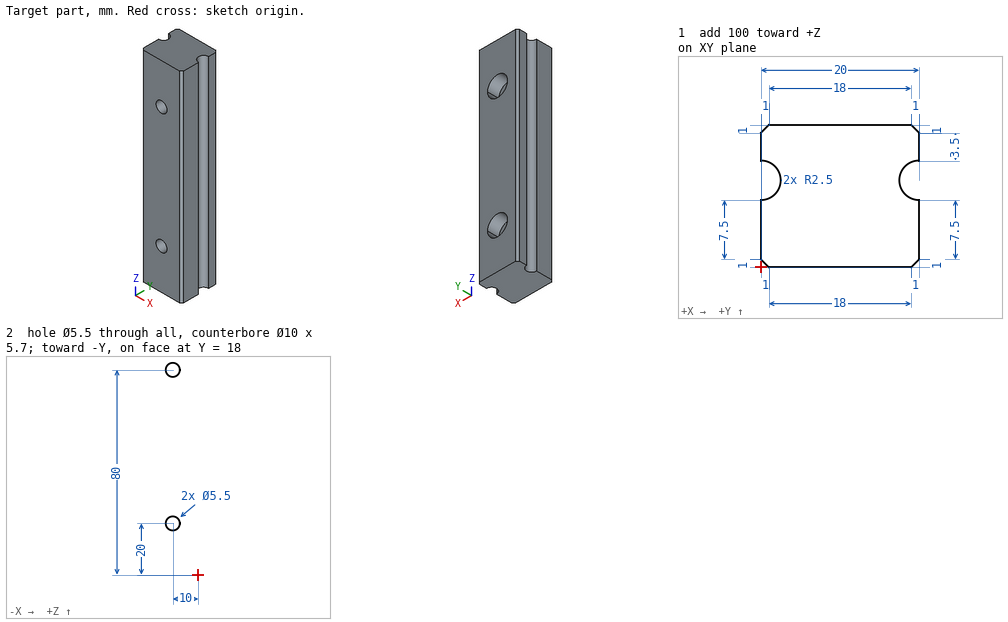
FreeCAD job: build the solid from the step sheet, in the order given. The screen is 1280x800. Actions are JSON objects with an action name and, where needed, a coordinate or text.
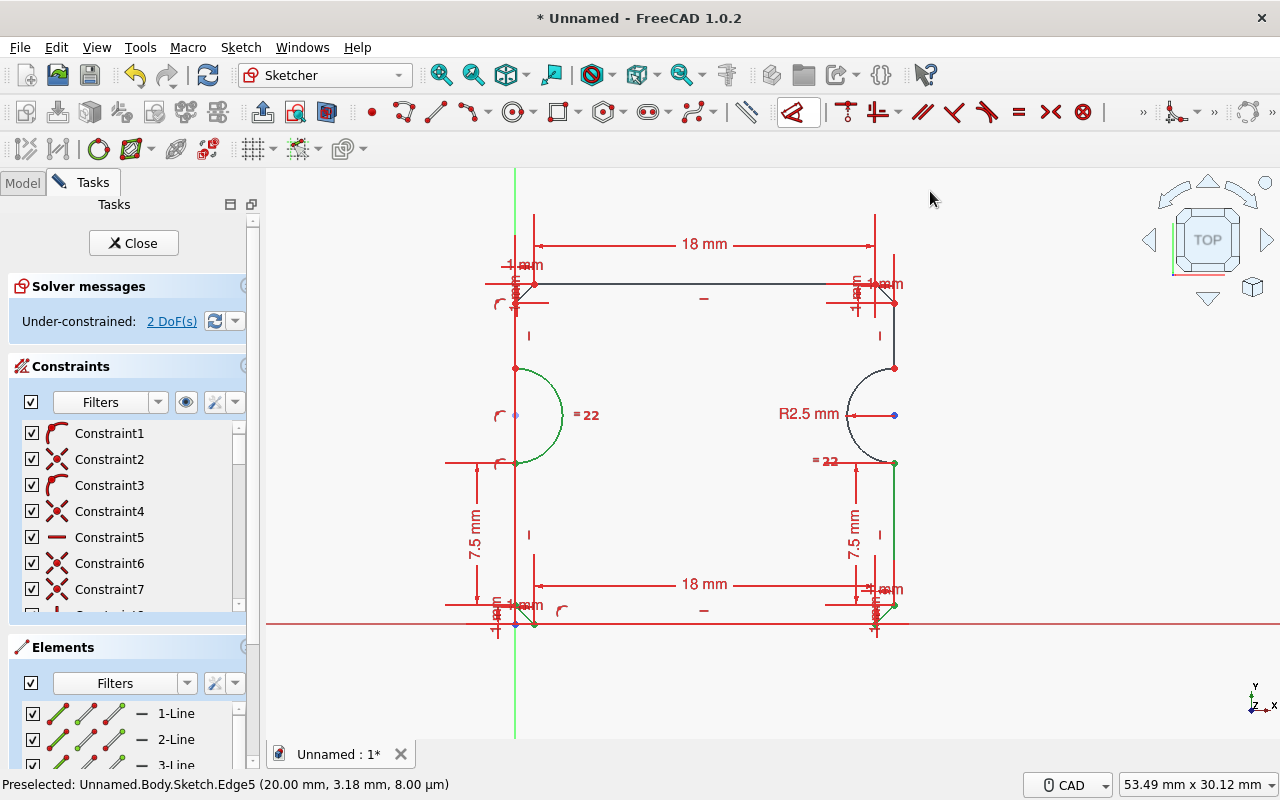
{"action": "left_click", "coordinate": [894, 349]}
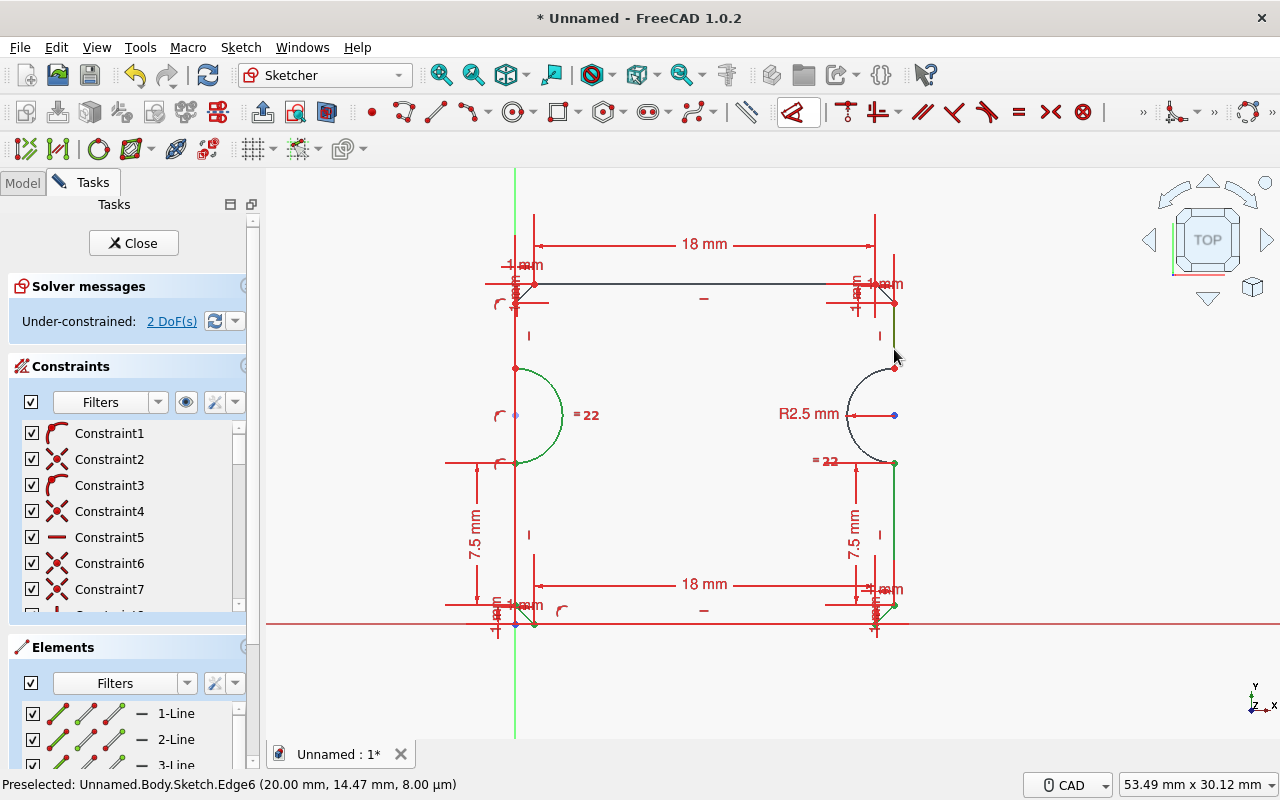
{"action": "left_click", "coordinate": [814, 112]}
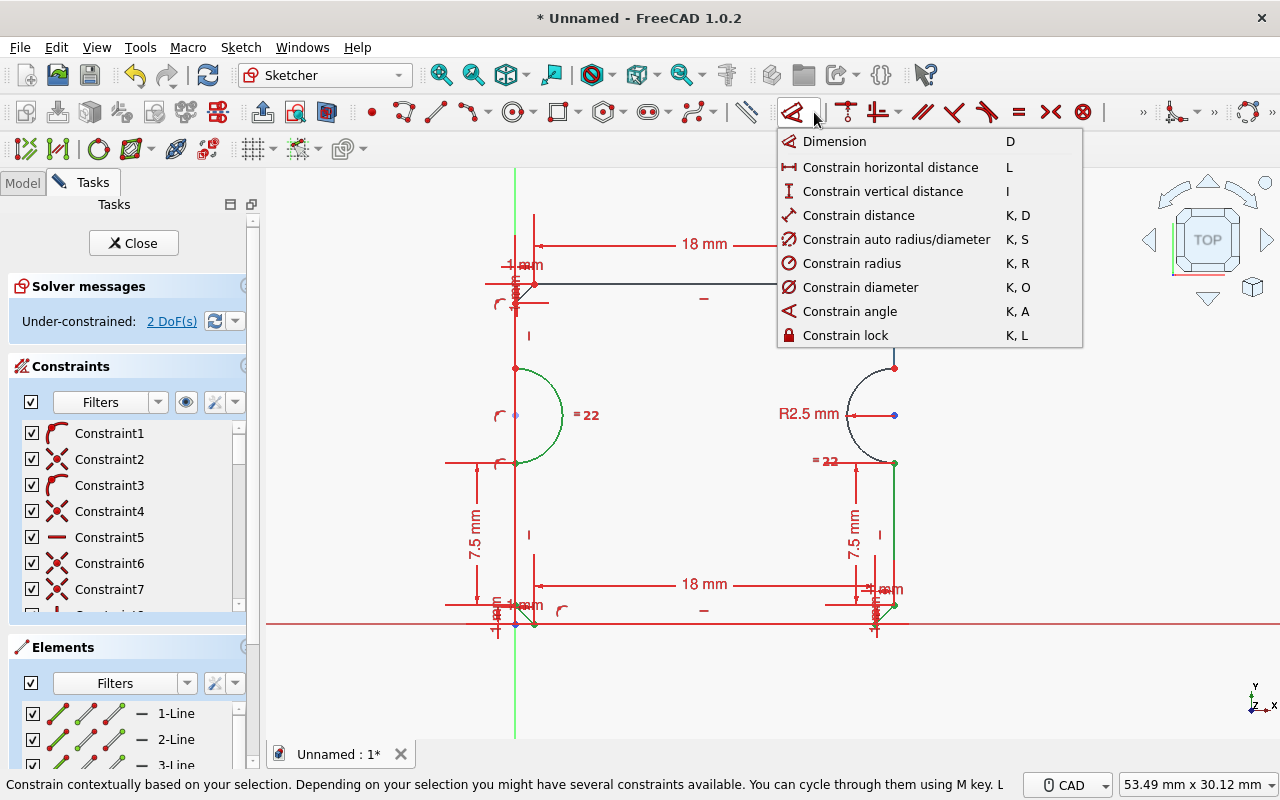
{"action": "left_click", "coordinate": [930, 191]}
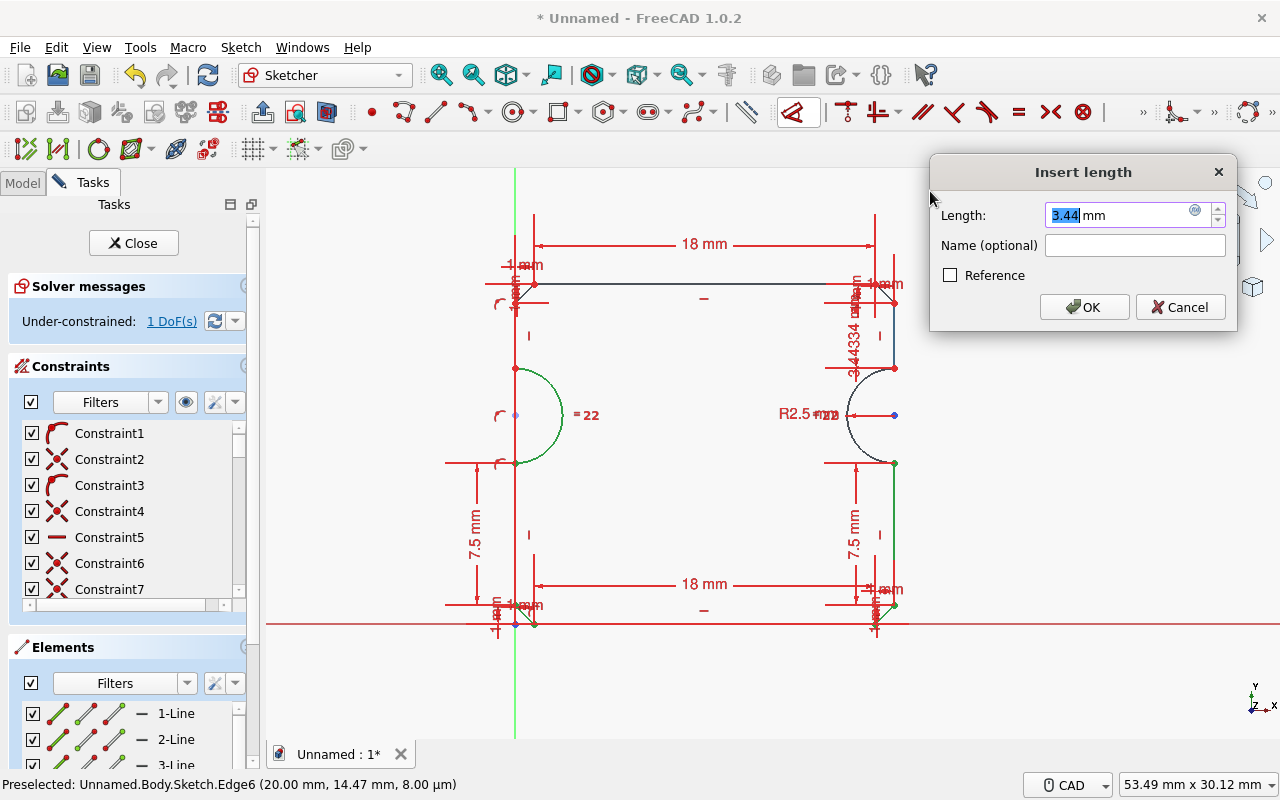
{"action": "type", "text": "3.5"}
{"action": "key", "text": "Return"}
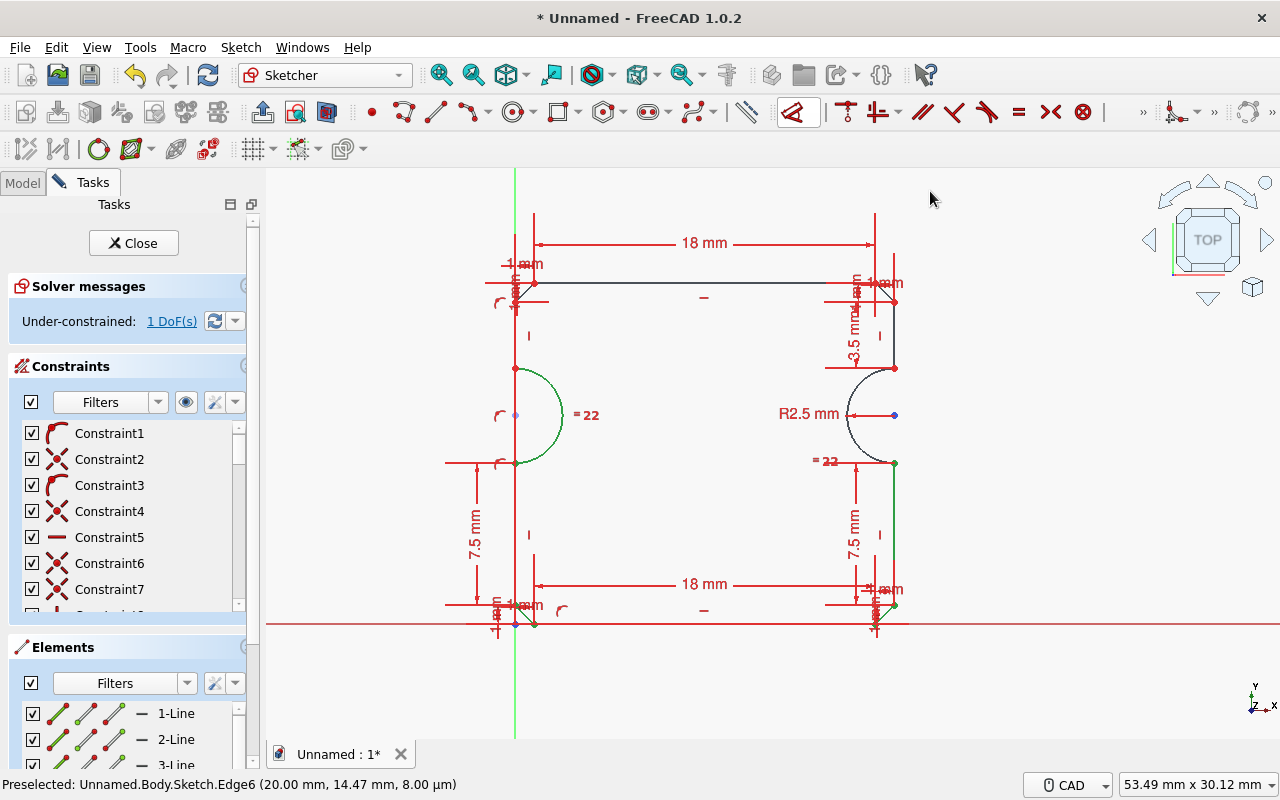
{"action": "left_click", "coordinate": [895, 416]}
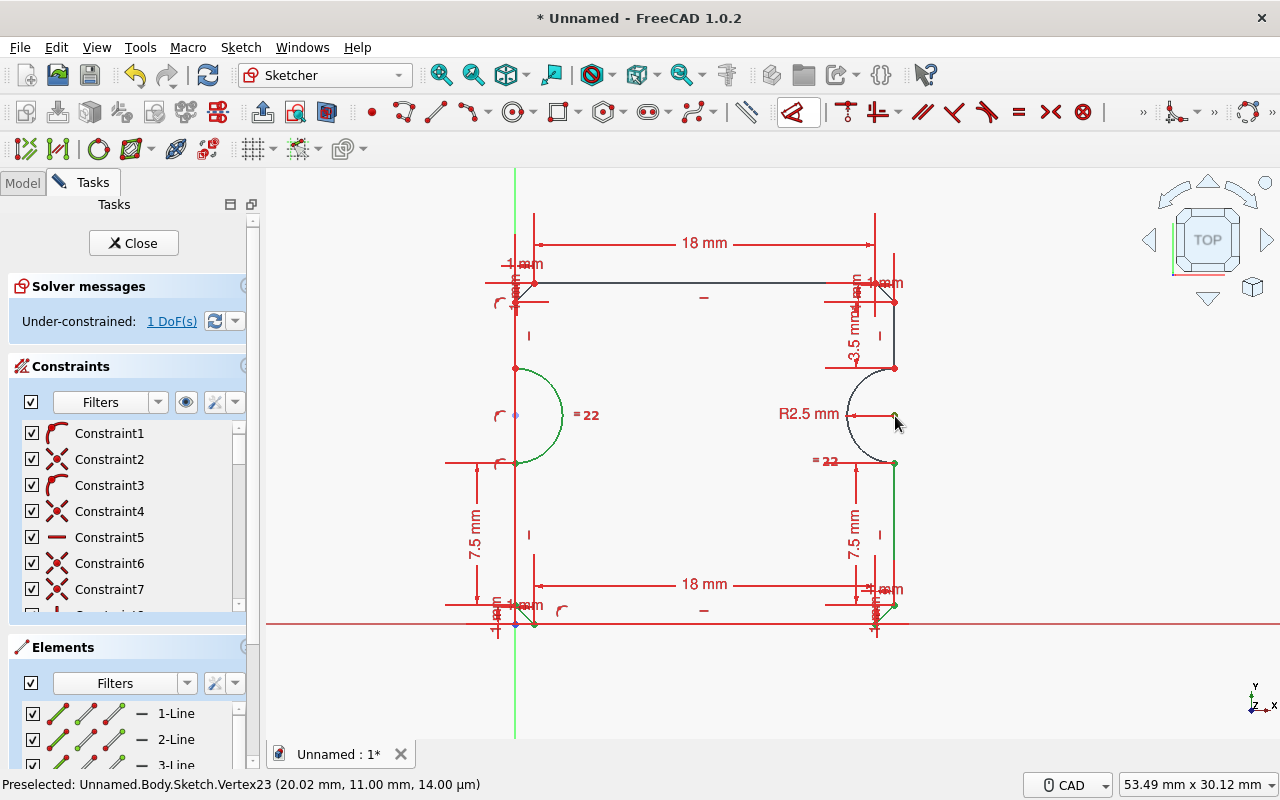
{"action": "left_click", "coordinate": [814, 112]}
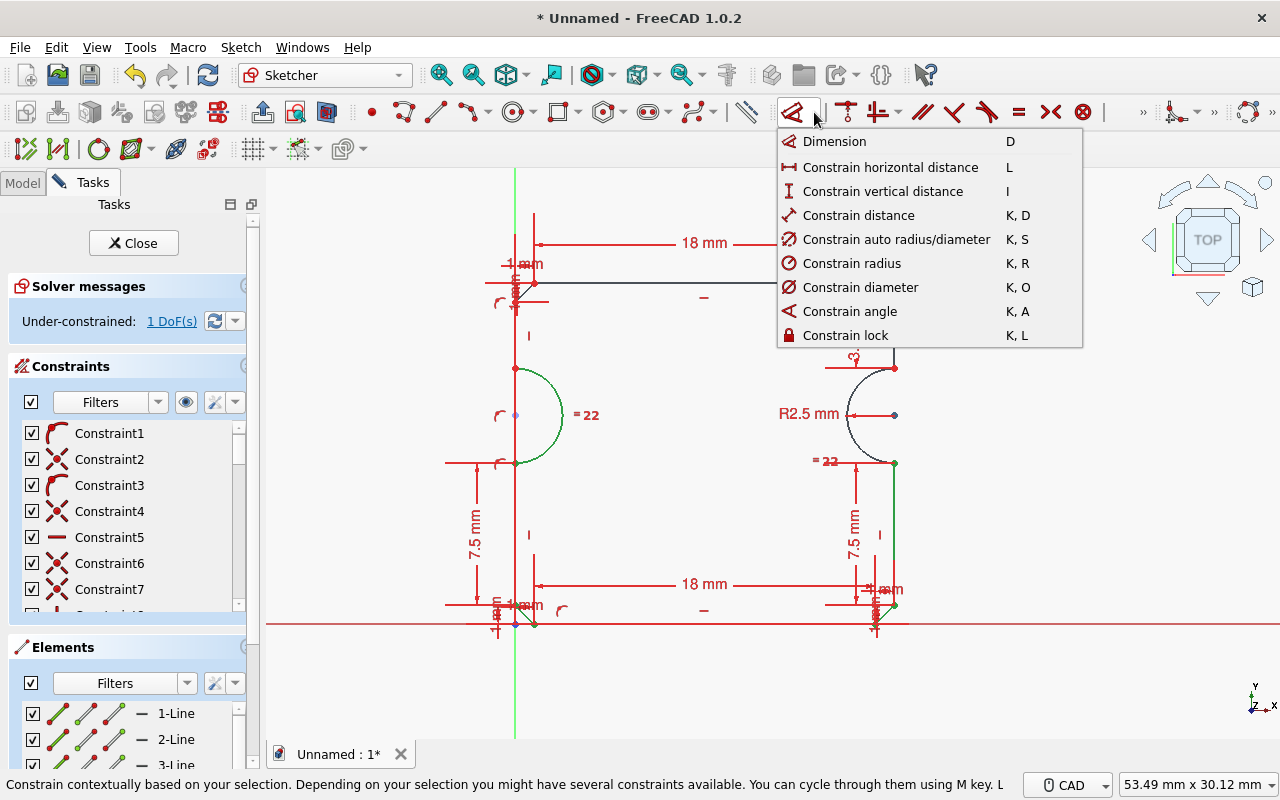
{"action": "left_click", "coordinate": [930, 167]}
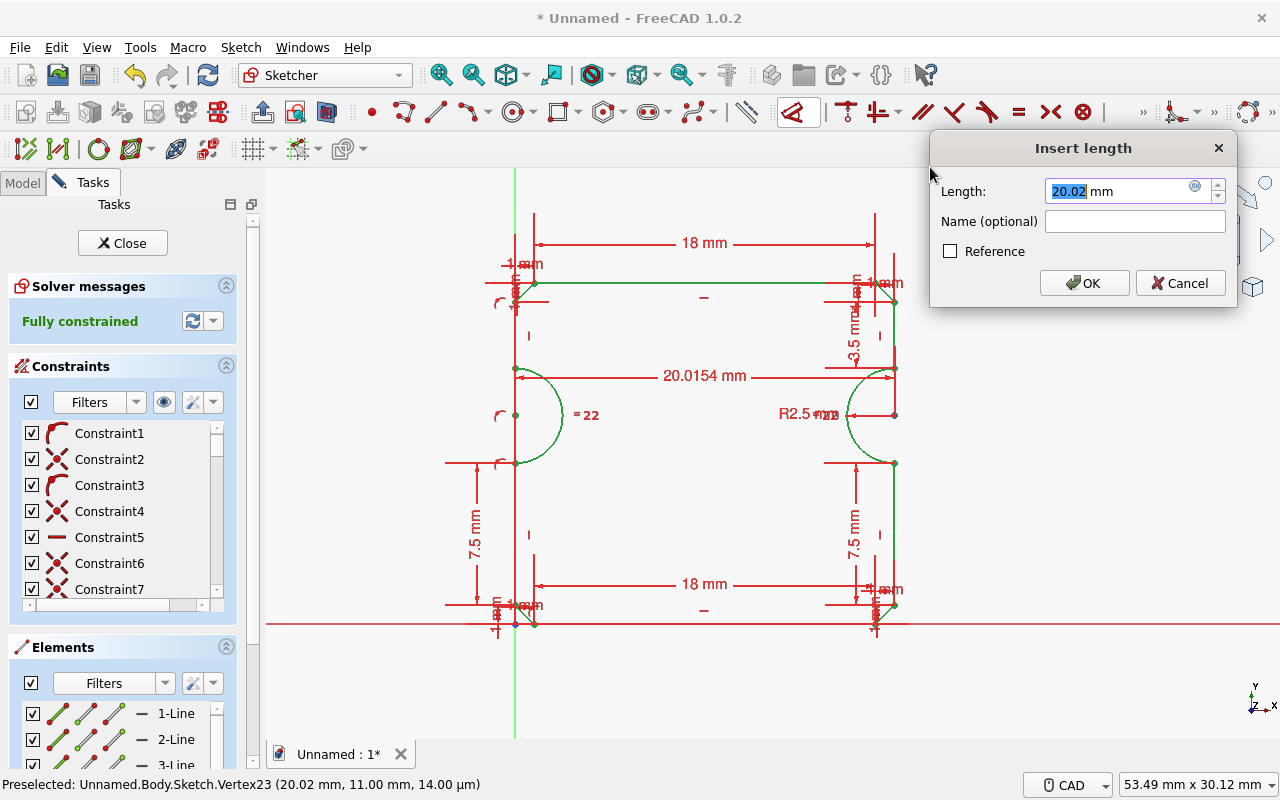
{"action": "type", "text": "20"}
{"action": "key", "text": "Return"}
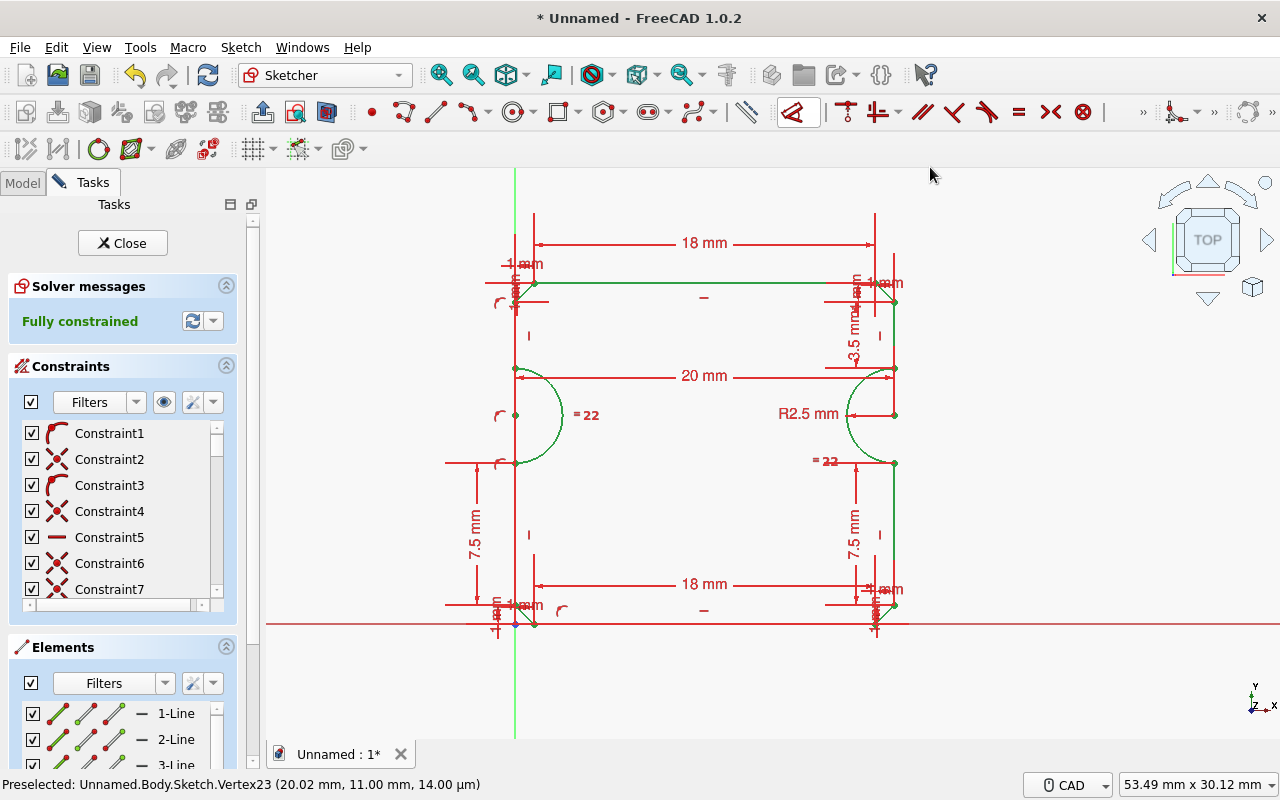
{"action": "left_click", "coordinate": [123, 243]}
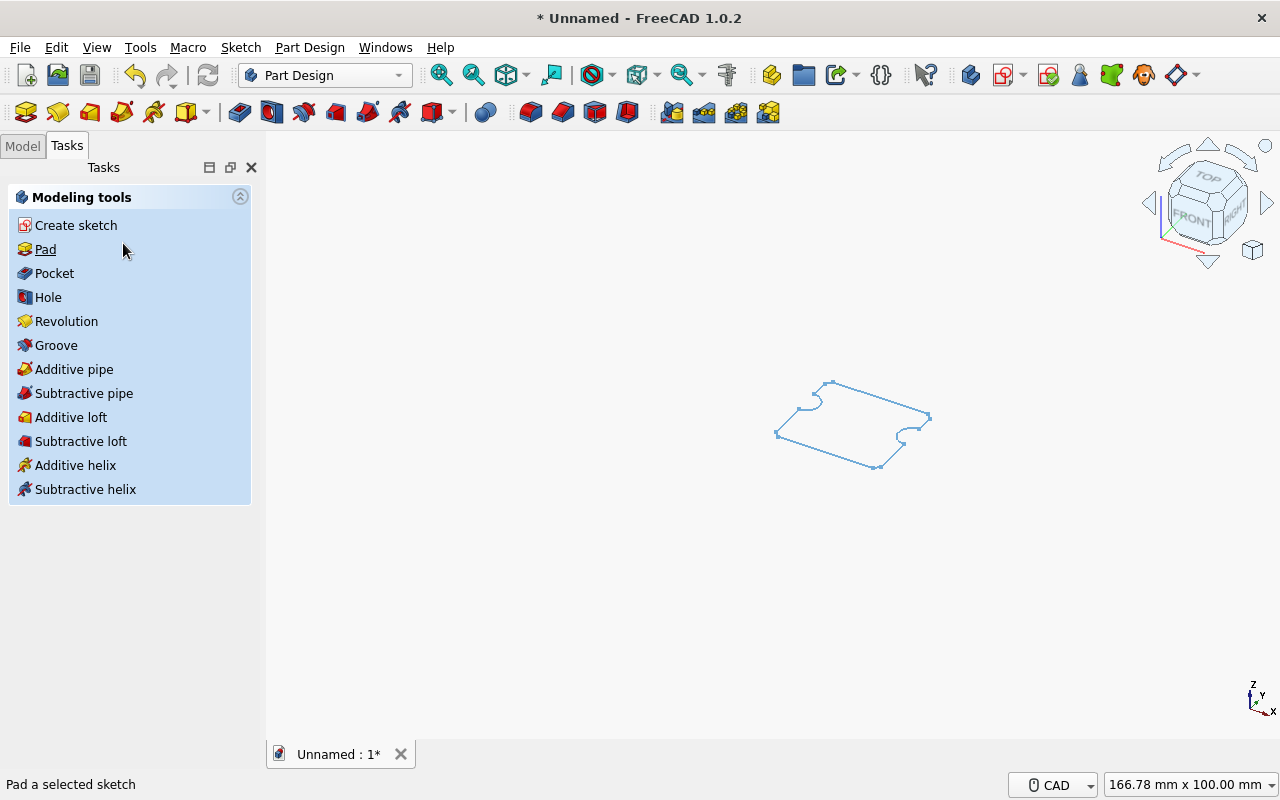
{"action": "left_click", "coordinate": [26, 112]}